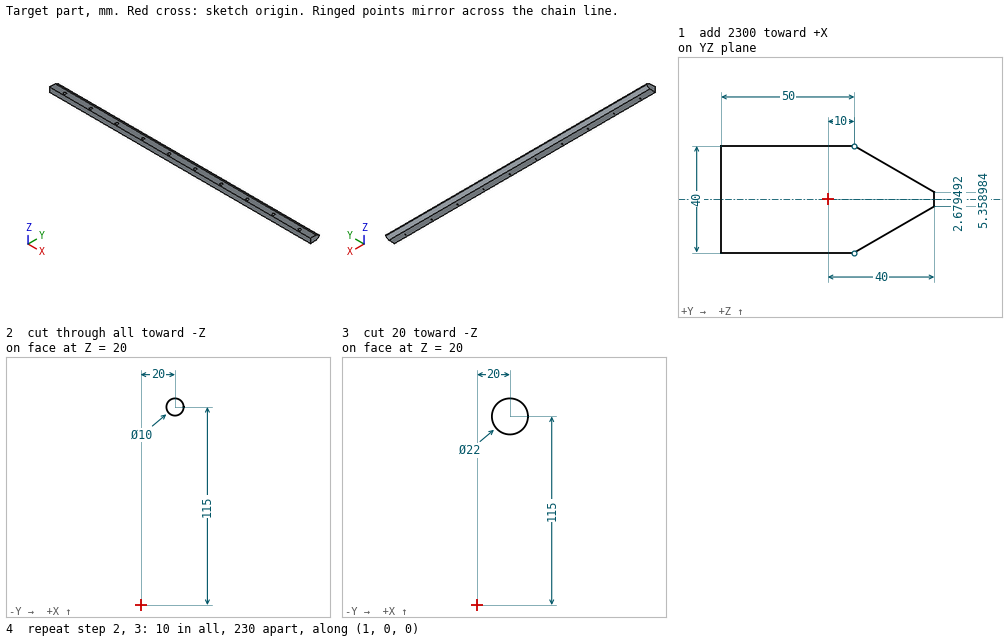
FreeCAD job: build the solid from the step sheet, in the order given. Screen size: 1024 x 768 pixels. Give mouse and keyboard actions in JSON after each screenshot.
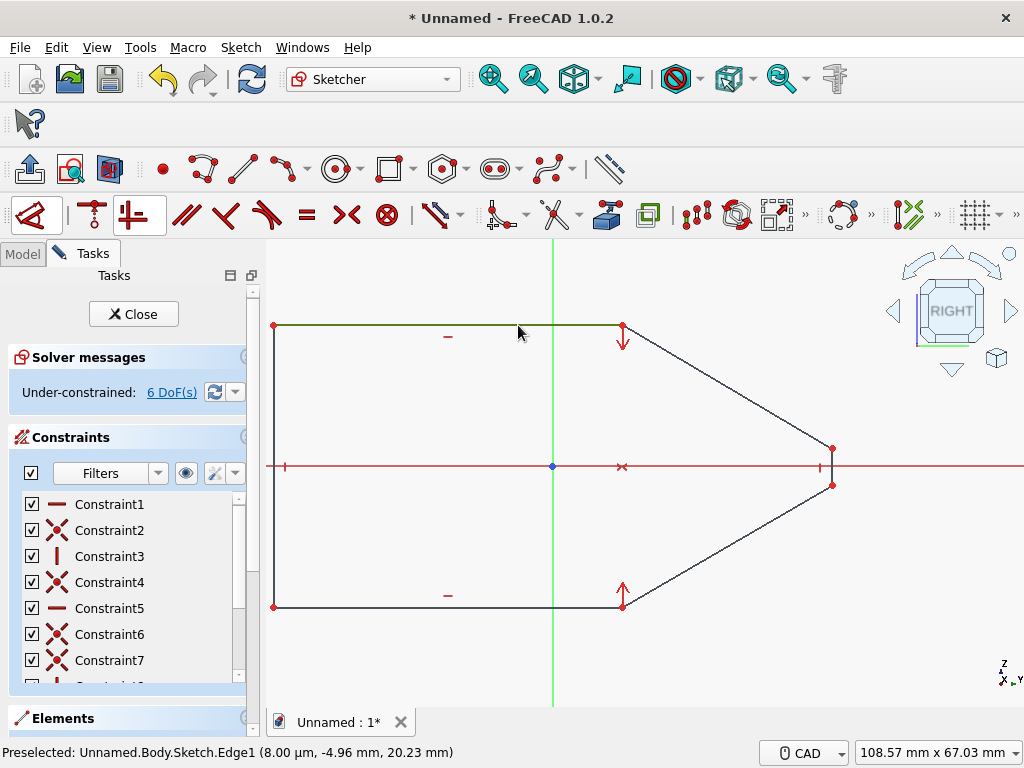
{"action": "key", "text": "l"}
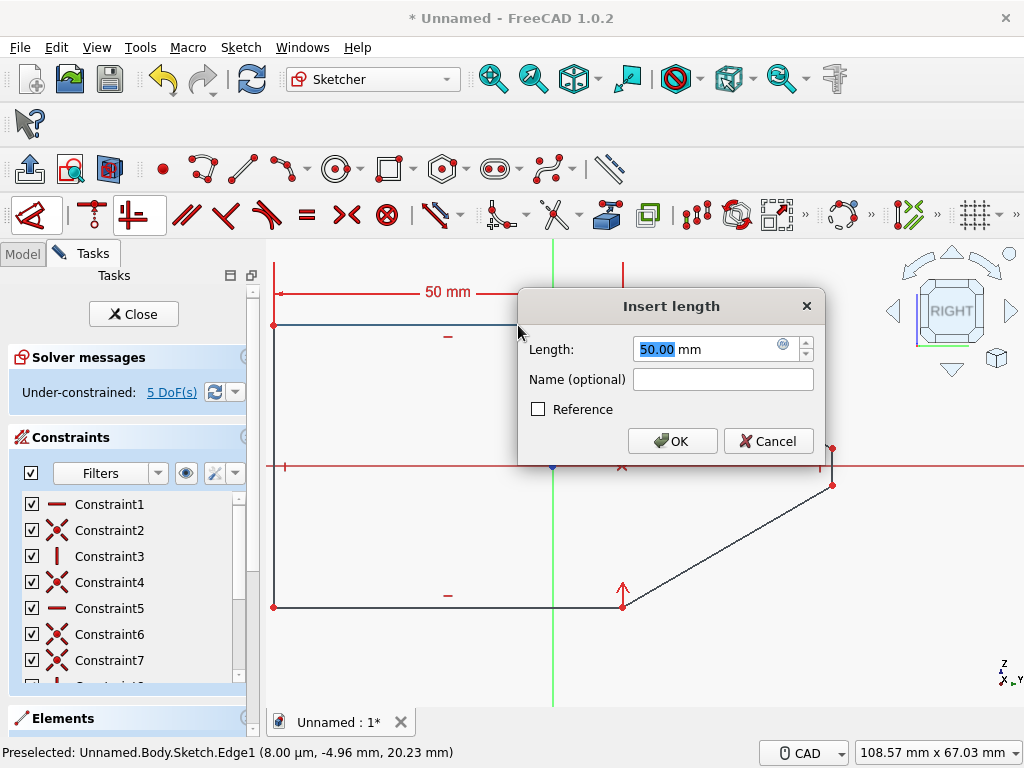
{"action": "type", "text": "50"}
{"action": "key", "text": "Return"}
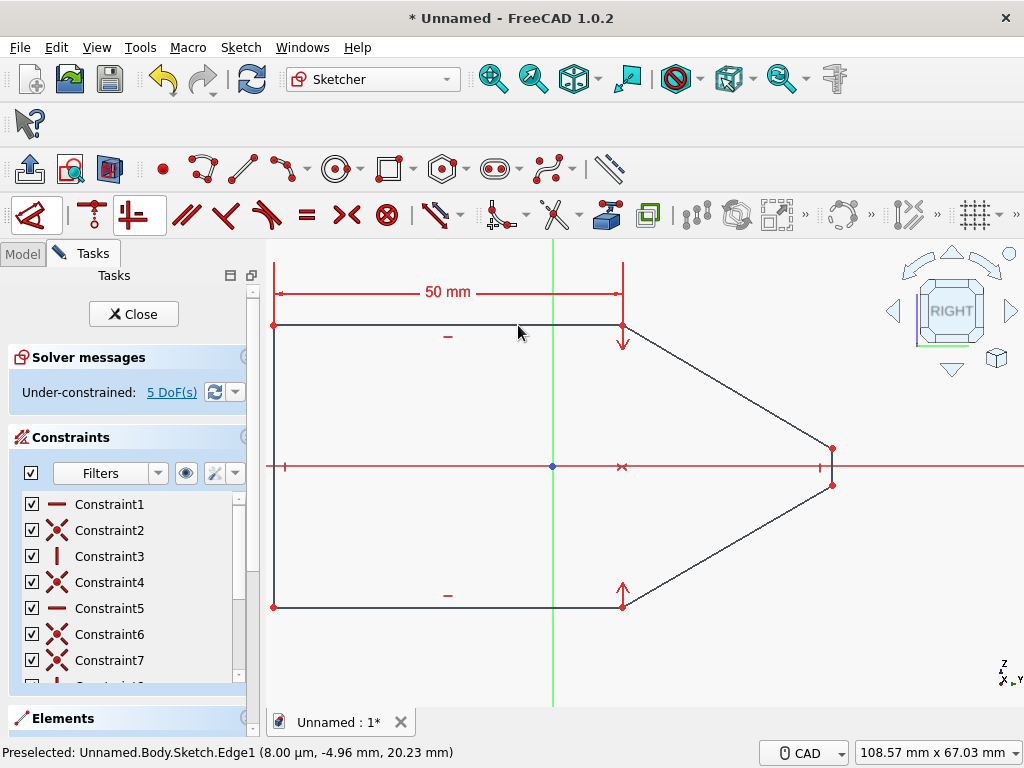
{"action": "scroll", "coordinate": [625, 487], "scroll_direction": "down", "scroll_amount": 2}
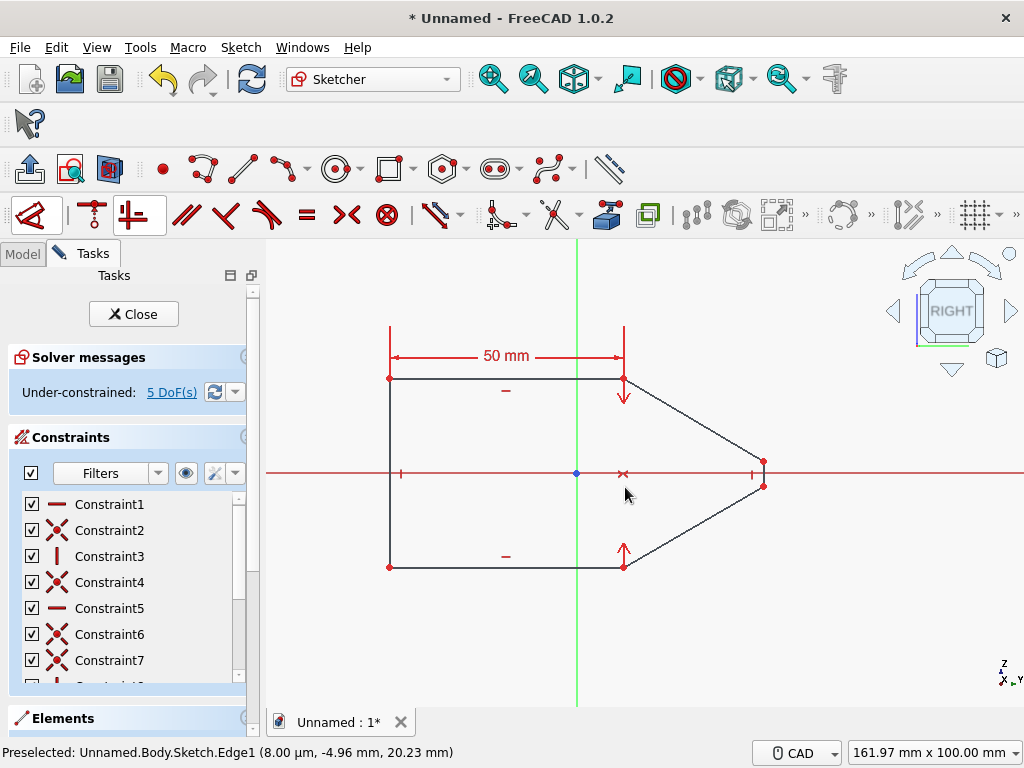
{"action": "left_click", "coordinate": [390, 435]}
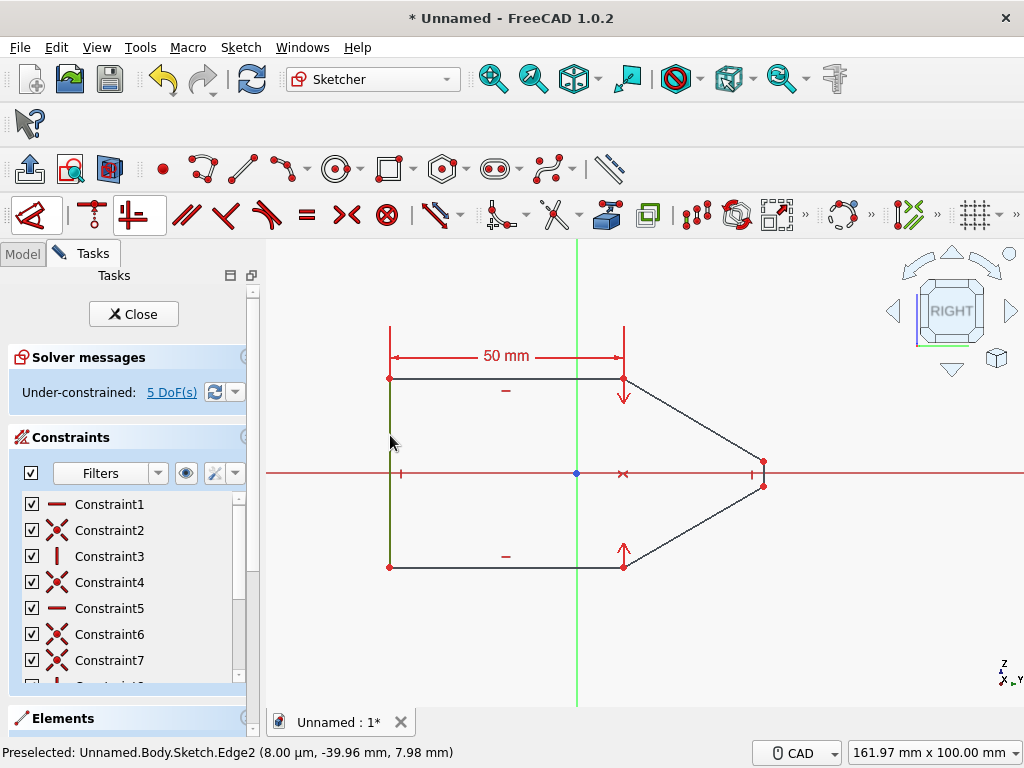
{"action": "key", "text": "i"}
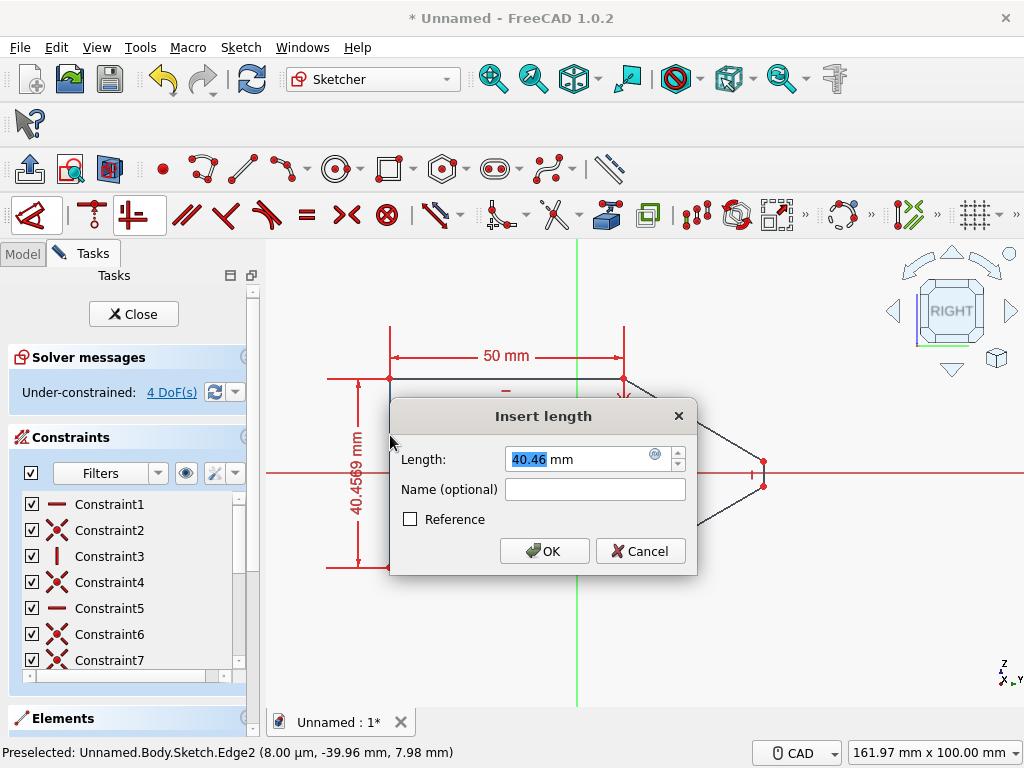
{"action": "type", "text": "40"}
{"action": "key", "text": "Return"}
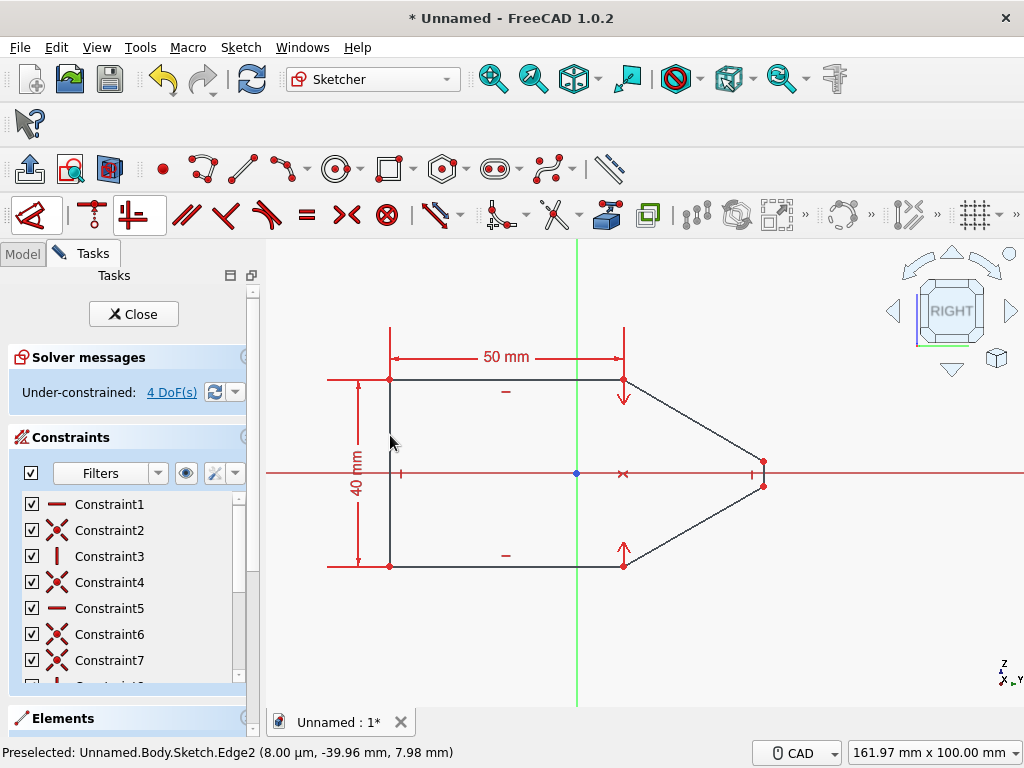
{"action": "left_click", "coordinate": [624, 380]}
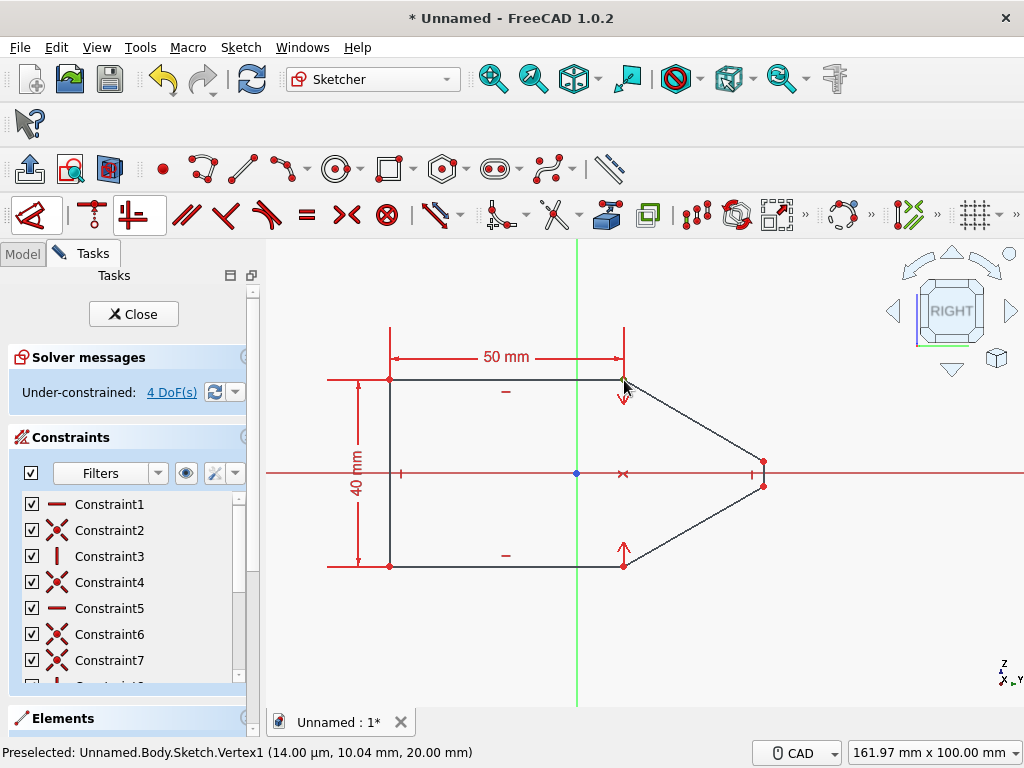
{"action": "key", "text": "l"}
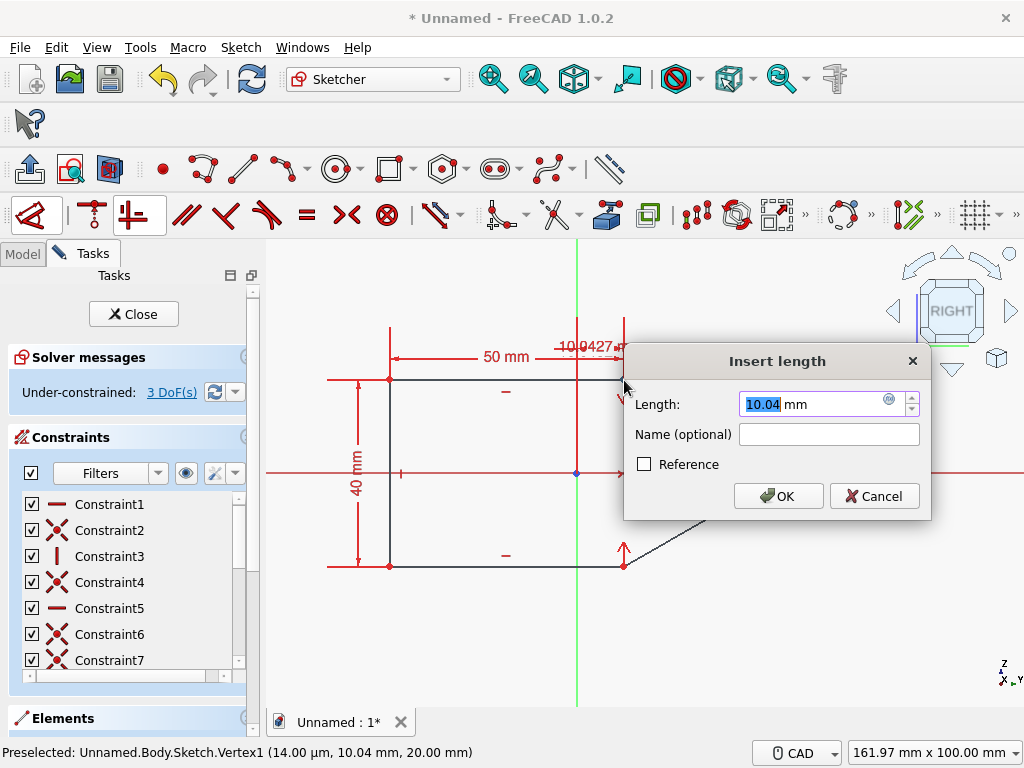
{"action": "type", "text": "10"}
{"action": "key", "text": "Return"}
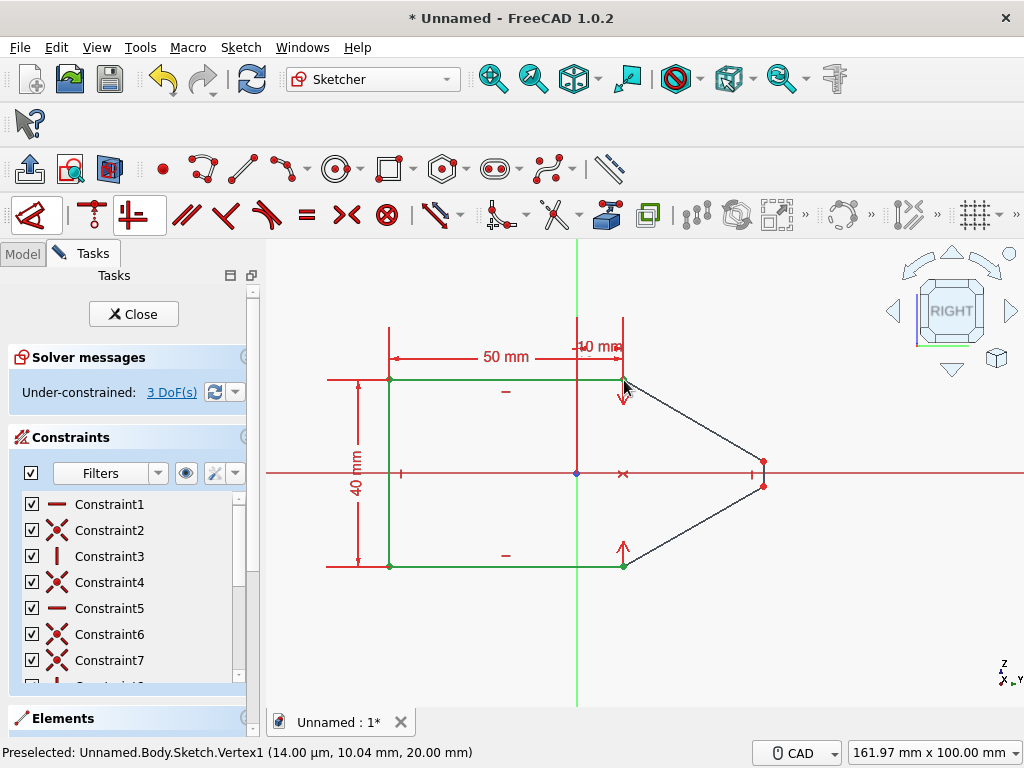
{"action": "left_click", "coordinate": [764, 487]}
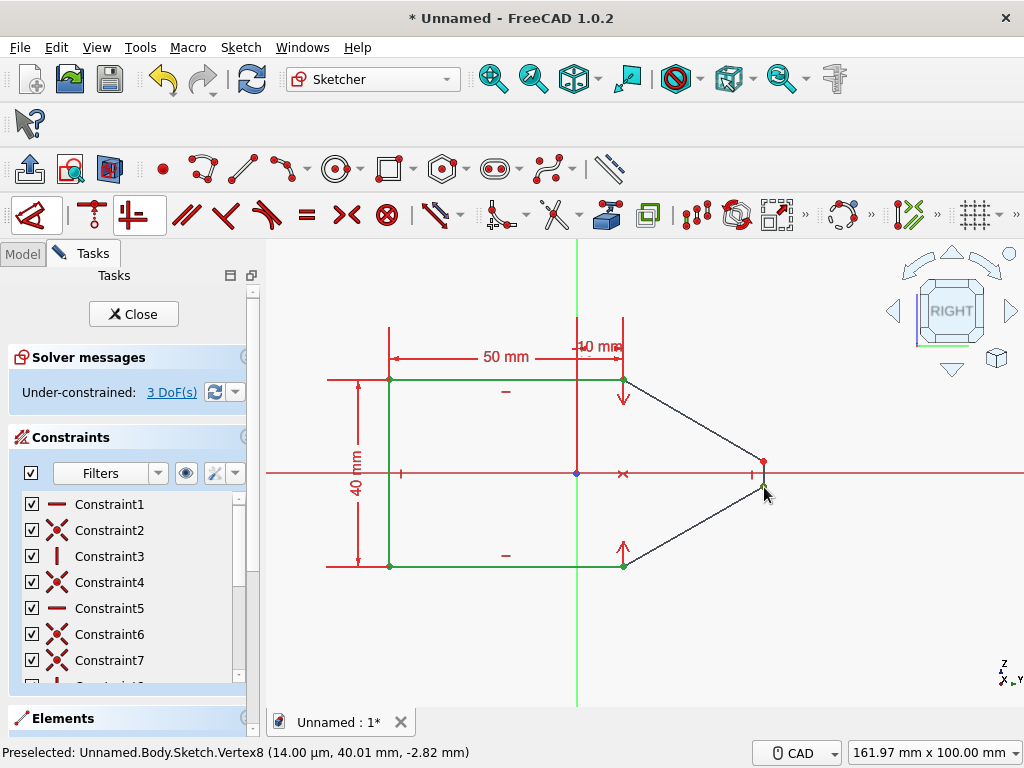
{"action": "key", "text": "l"}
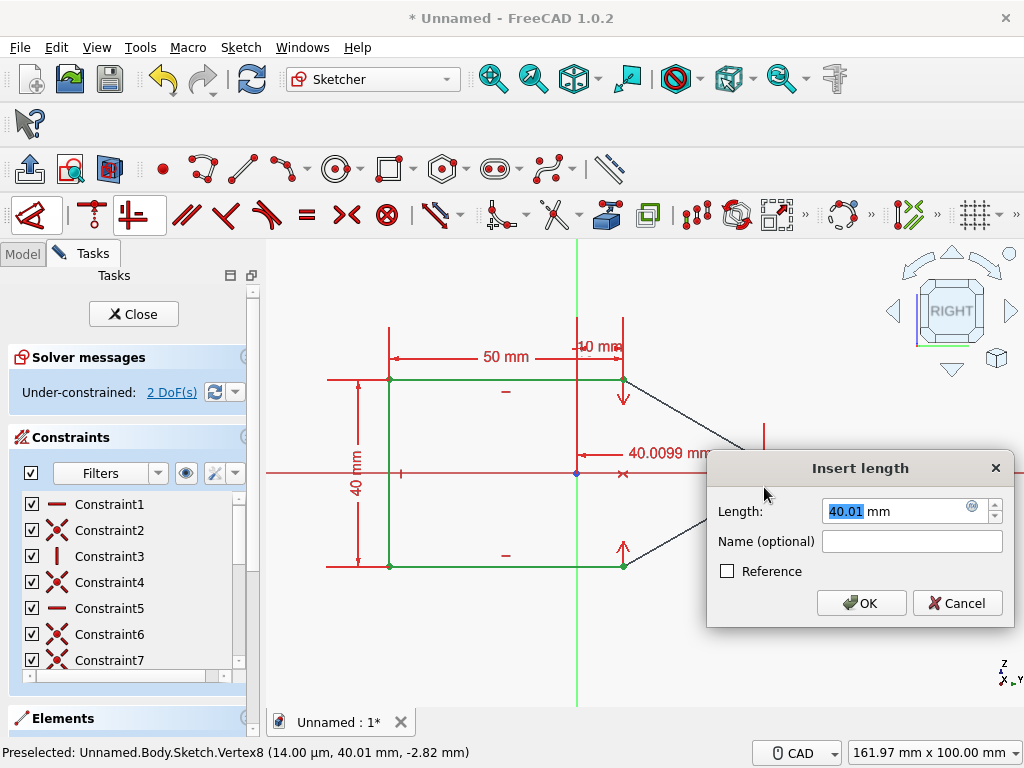
{"action": "type", "text": "40"}
{"action": "key", "text": "Return"}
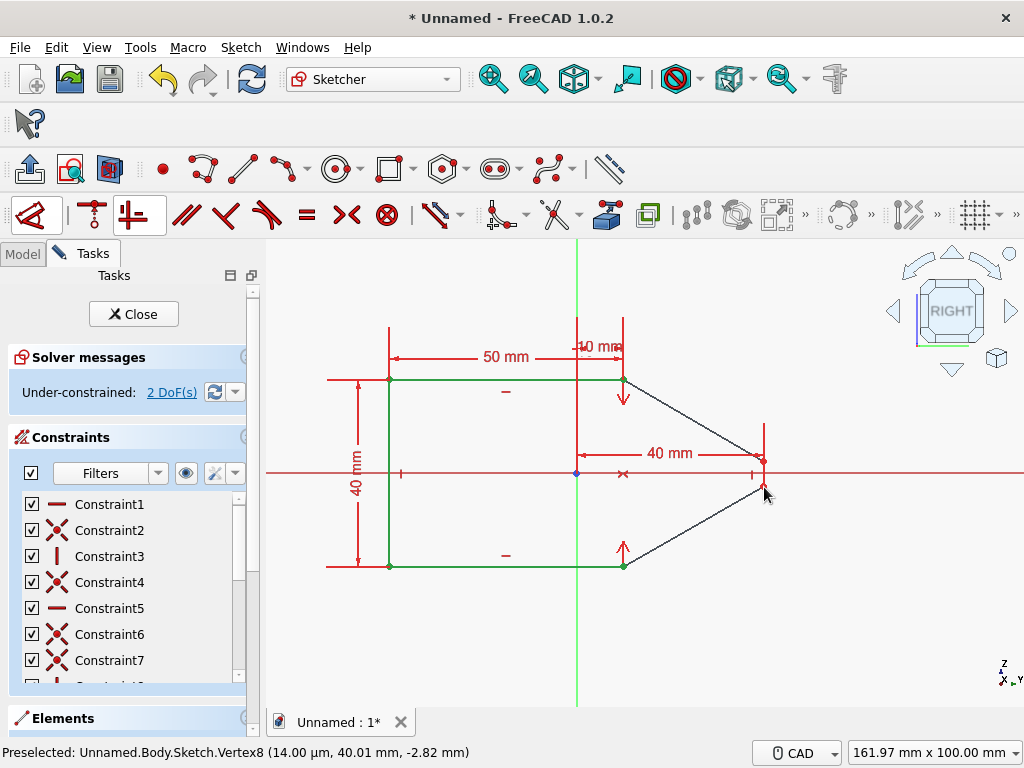
{"action": "scroll", "coordinate": [764, 477], "scroll_direction": "up", "scroll_amount": 3}